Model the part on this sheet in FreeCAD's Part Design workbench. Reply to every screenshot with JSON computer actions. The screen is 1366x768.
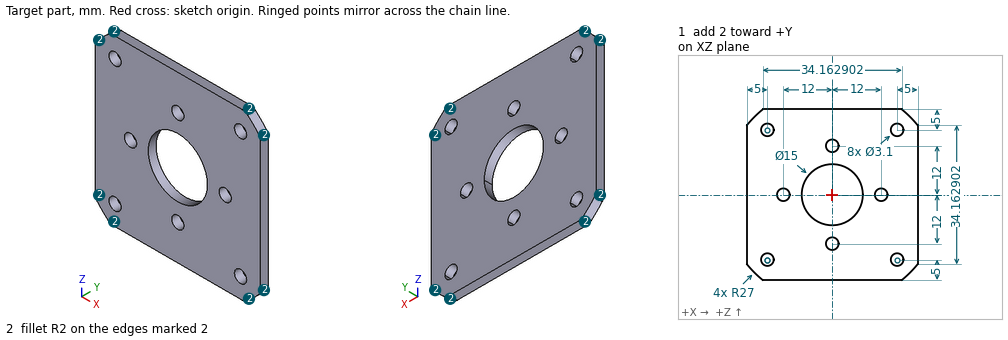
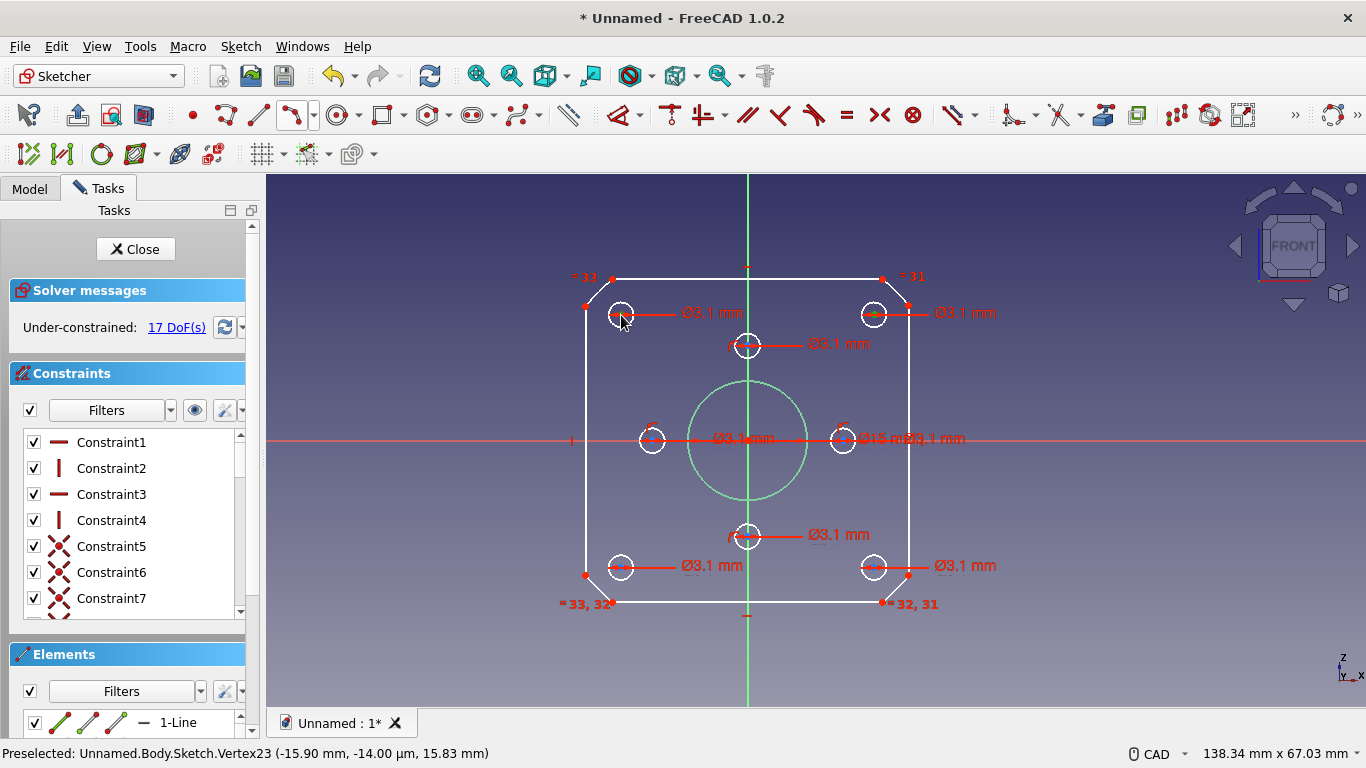
{"action": "left_click", "coordinate": [724, 116]}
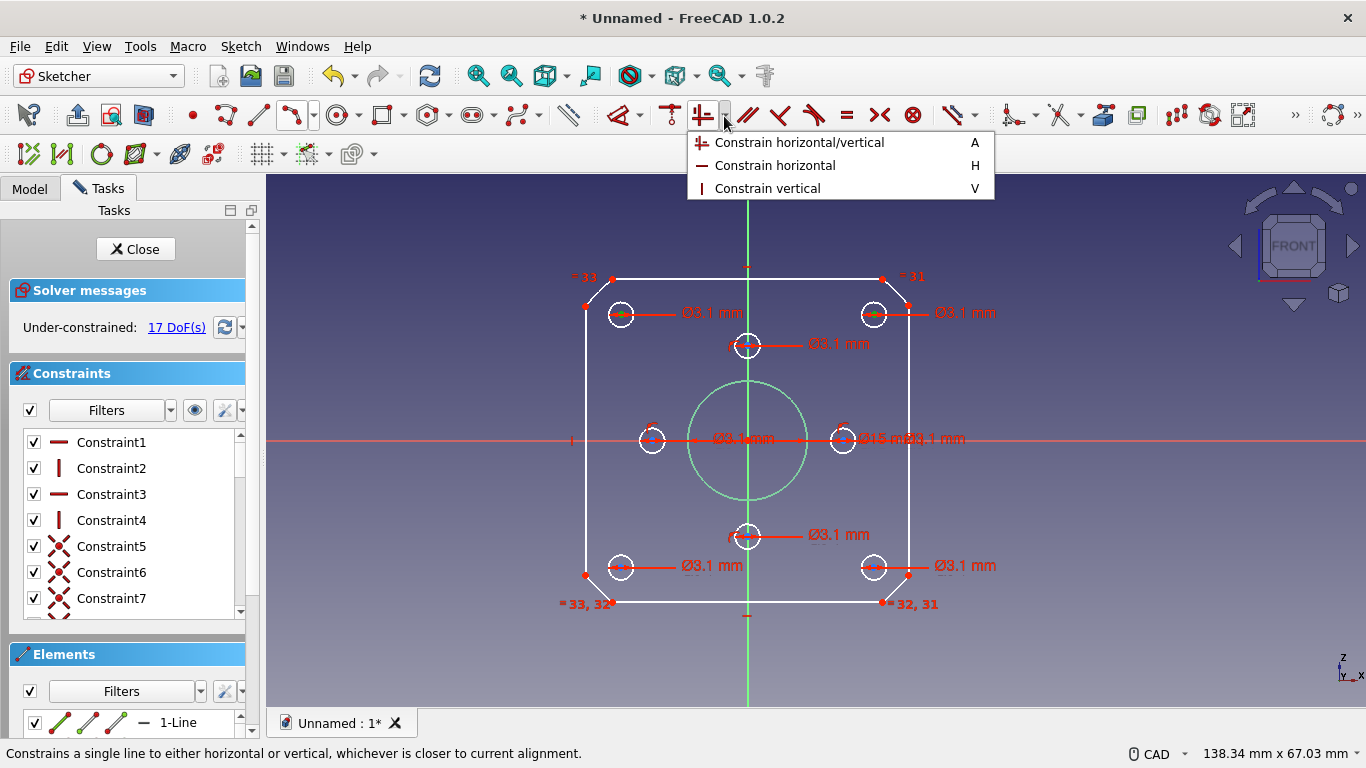
{"action": "left_click", "coordinate": [841, 166]}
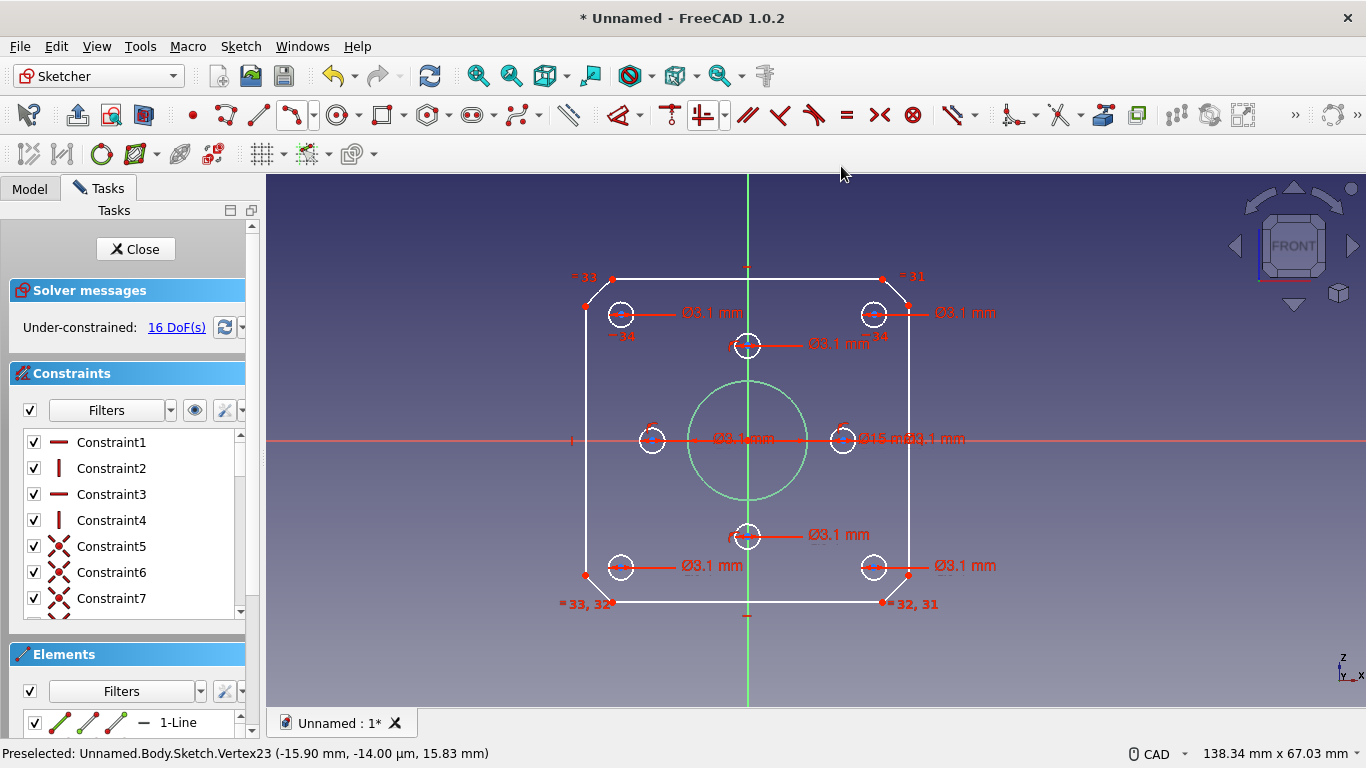
{"action": "left_click", "coordinate": [874, 315]}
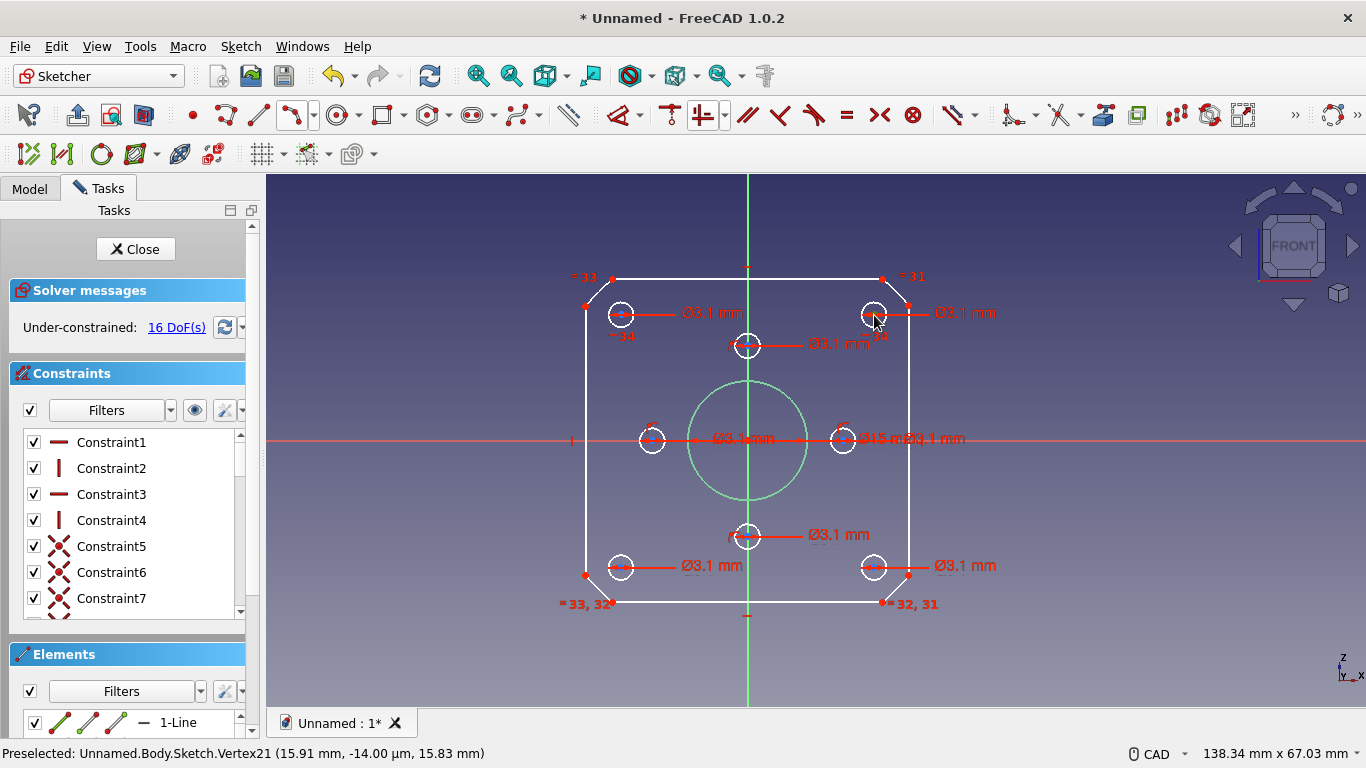
{"action": "left_click", "coordinate": [874, 568]}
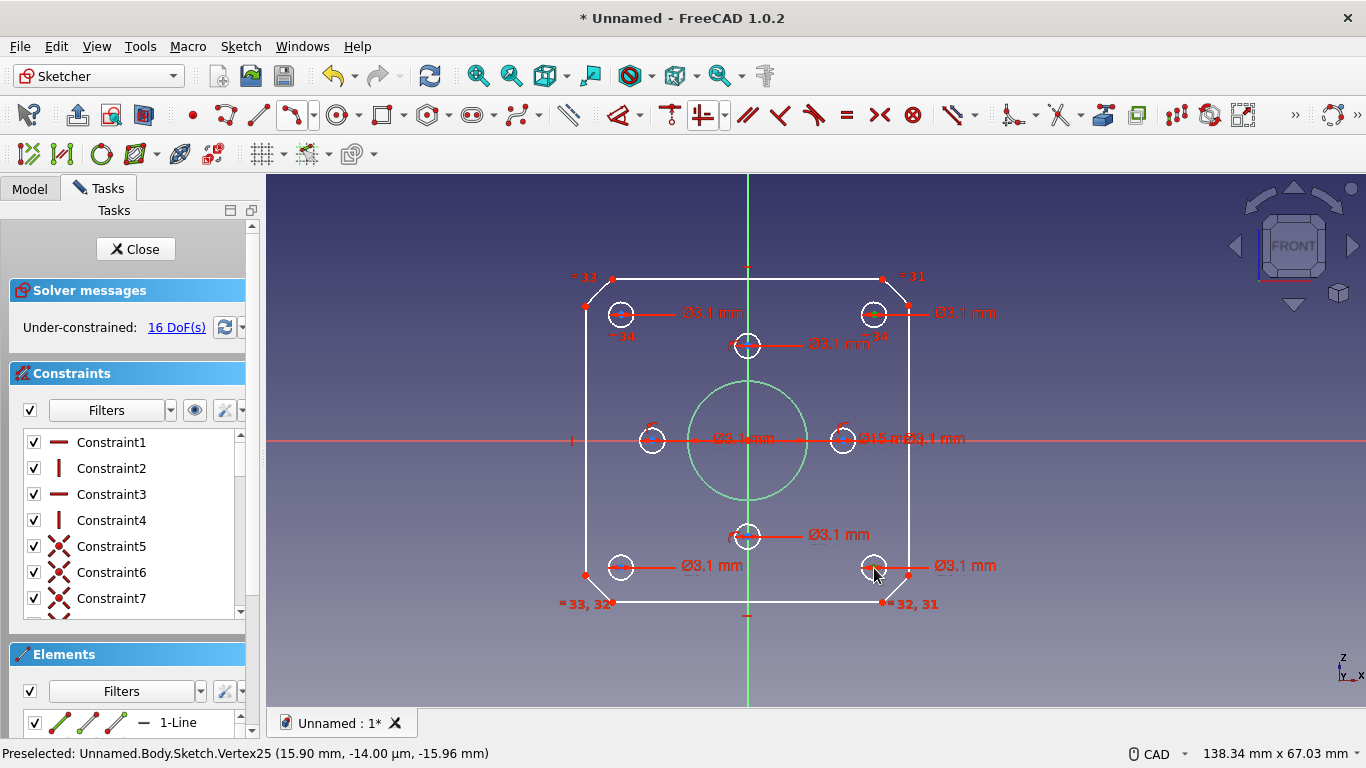
{"action": "left_click", "coordinate": [724, 116]}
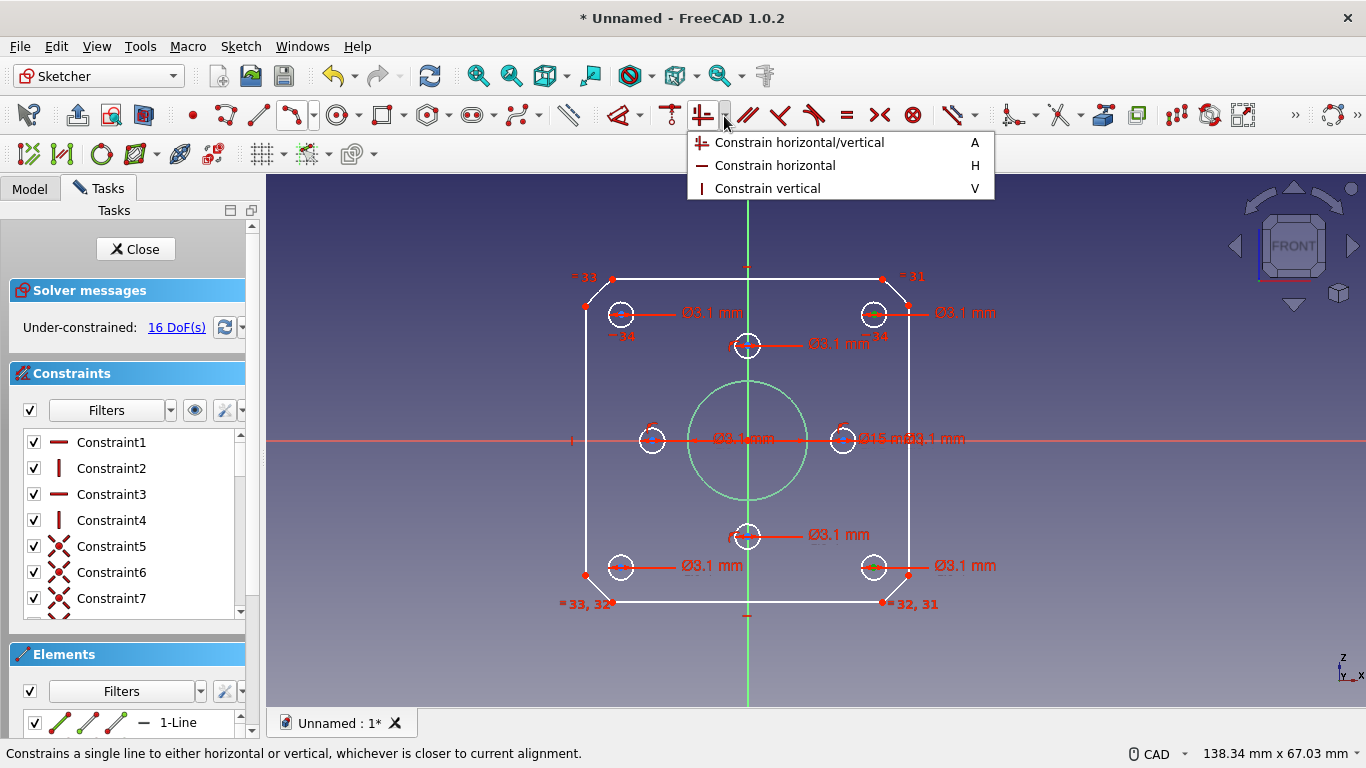
{"action": "left_click", "coordinate": [841, 188]}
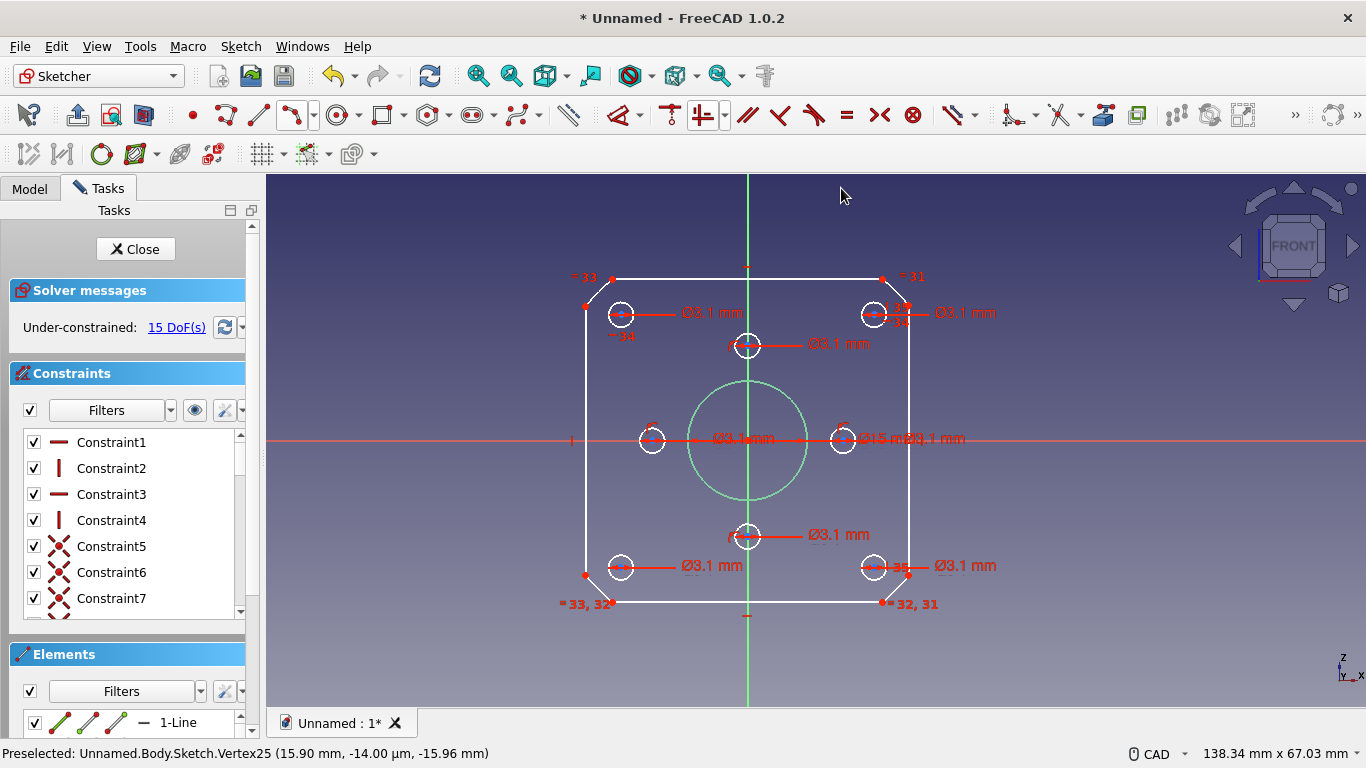
{"action": "left_click", "coordinate": [621, 315]}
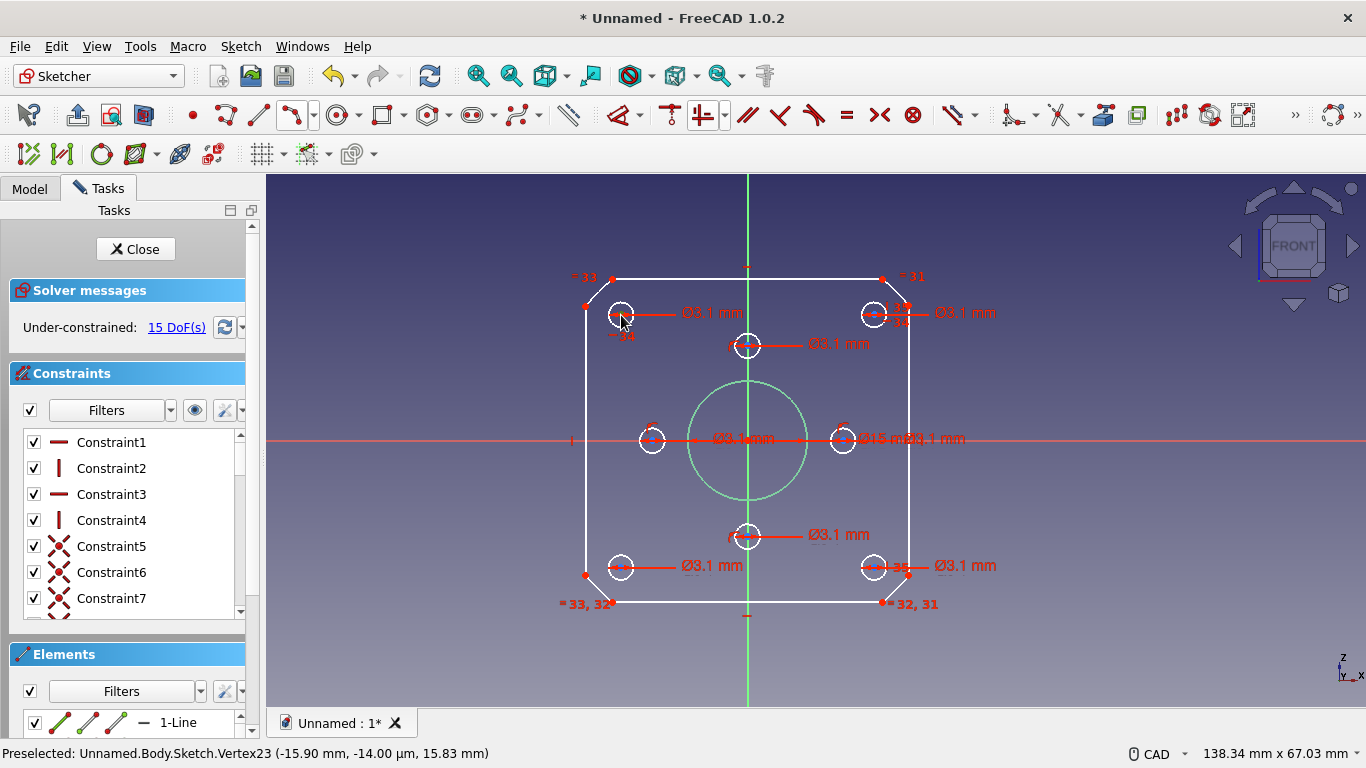
{"action": "left_click", "coordinate": [621, 568]}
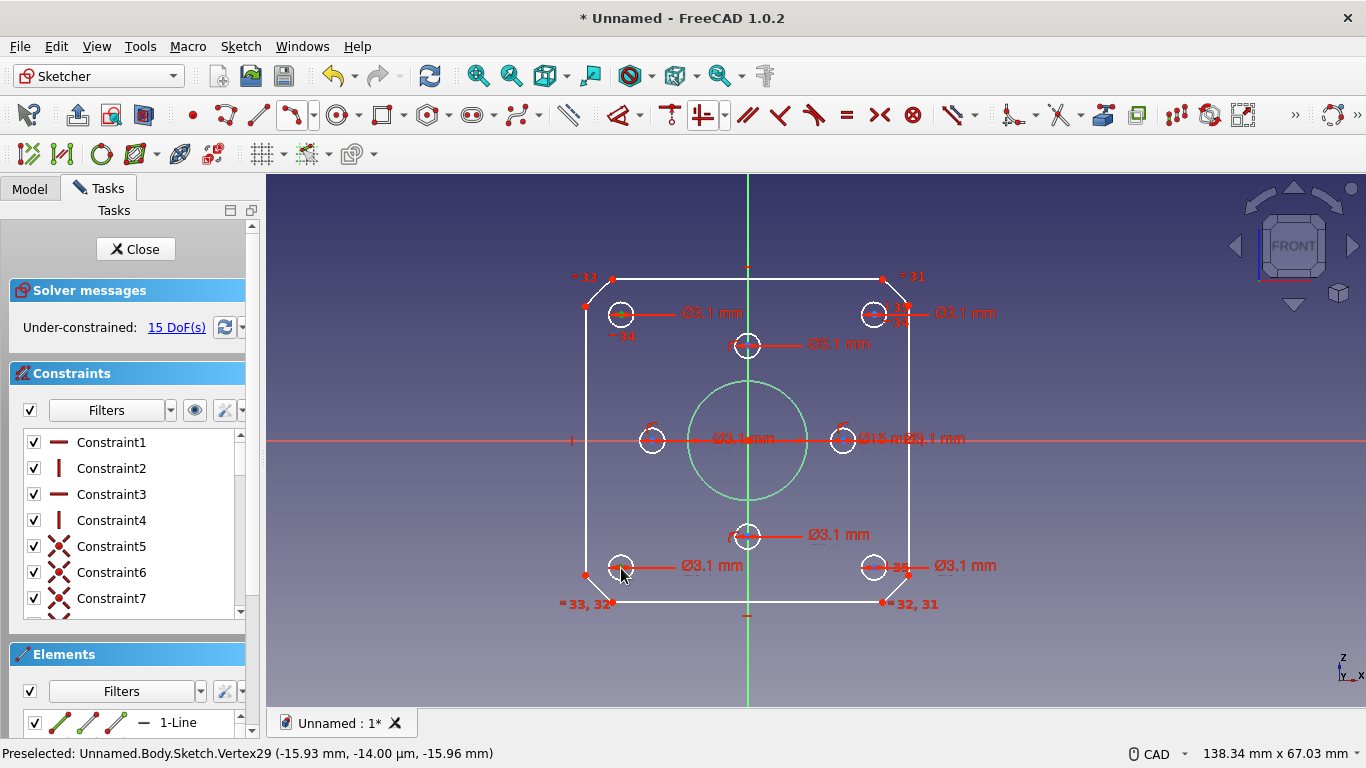
{"action": "left_click", "coordinate": [359, 441]}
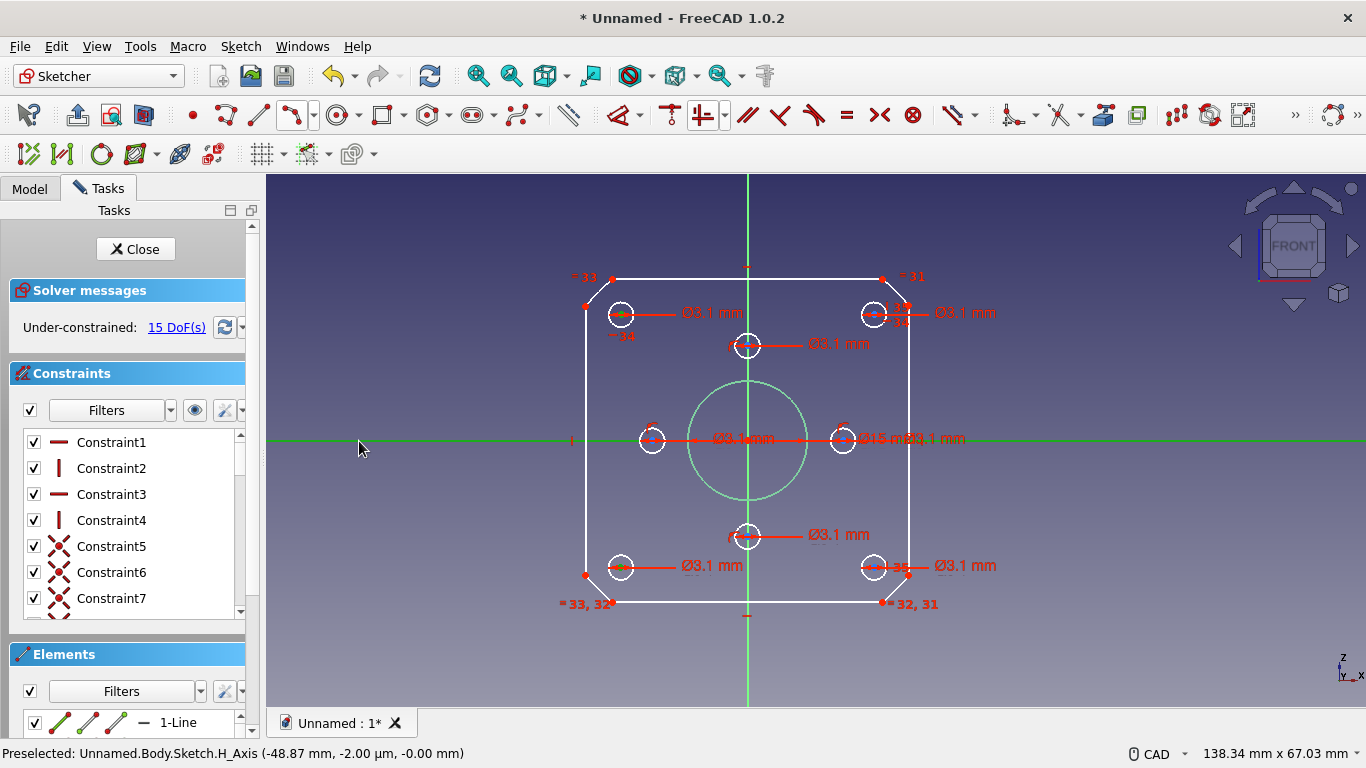
{"action": "left_click", "coordinate": [880, 116]}